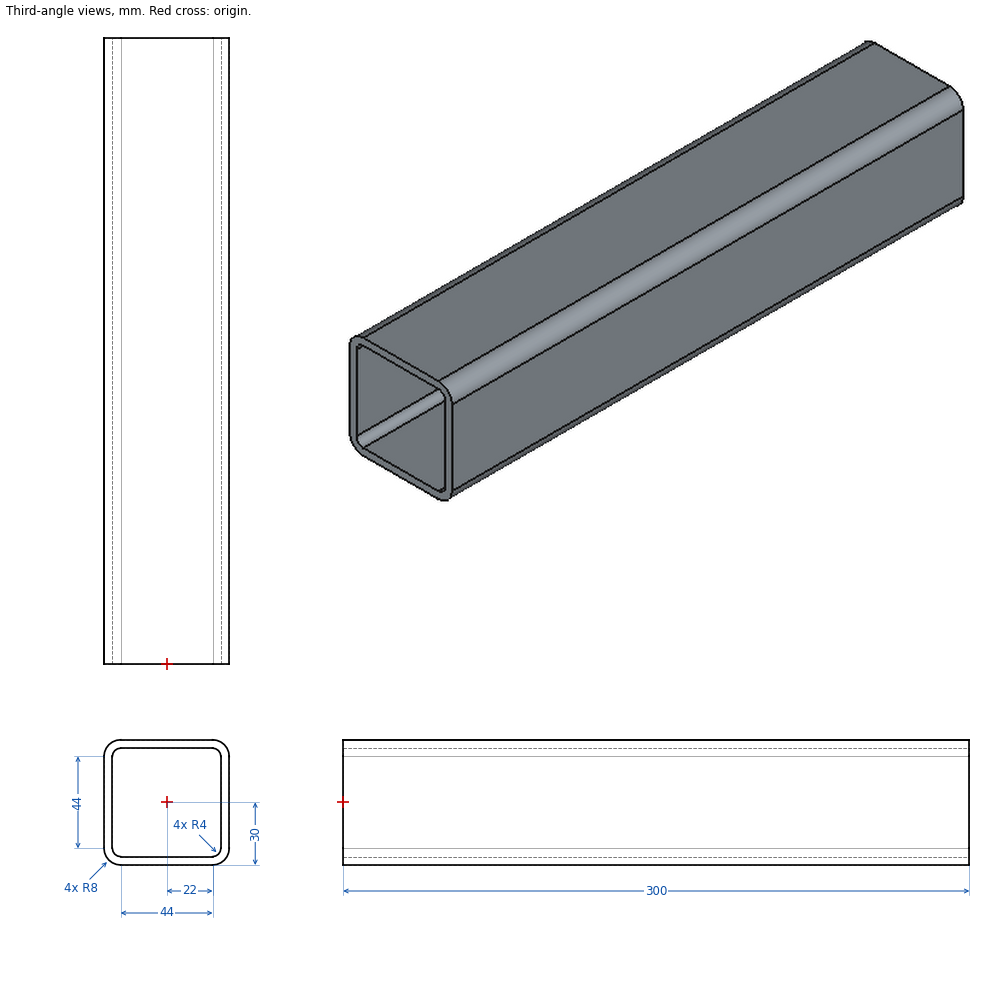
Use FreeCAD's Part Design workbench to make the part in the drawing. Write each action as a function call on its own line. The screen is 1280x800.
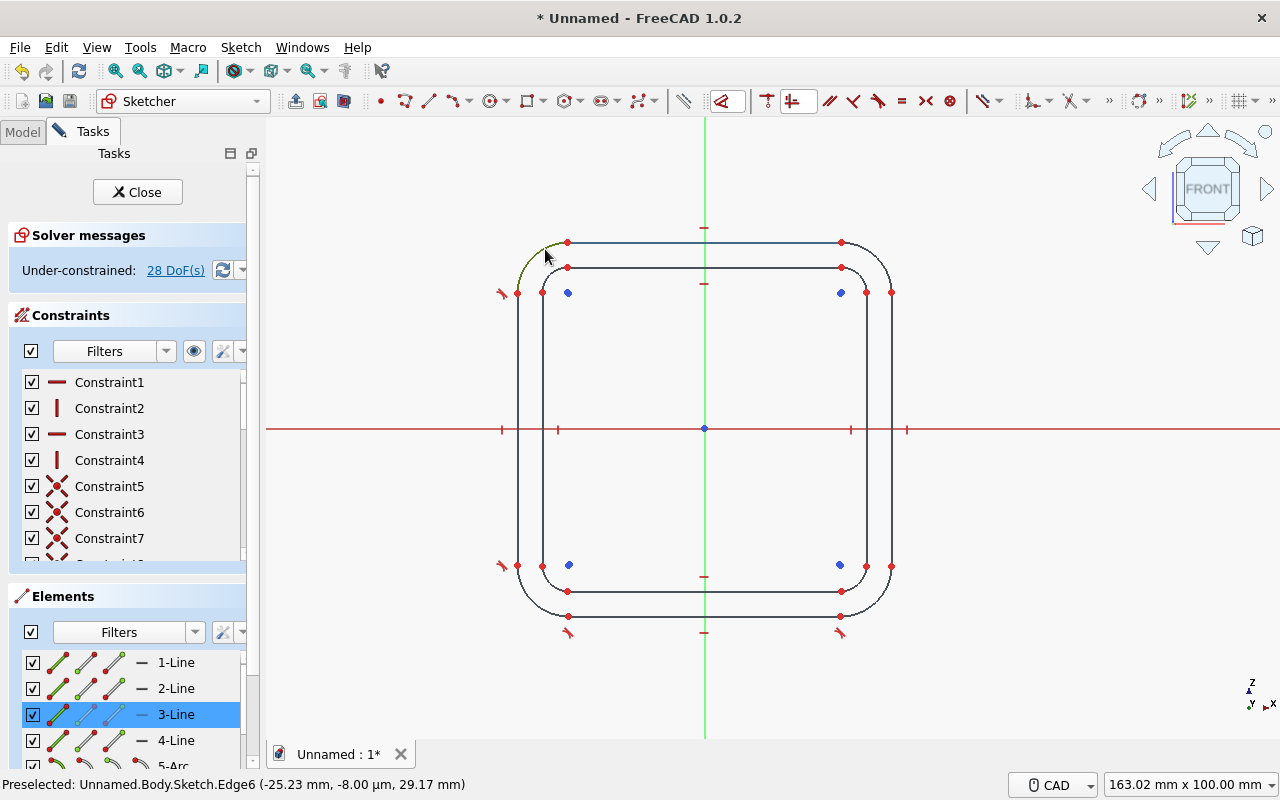
key(t)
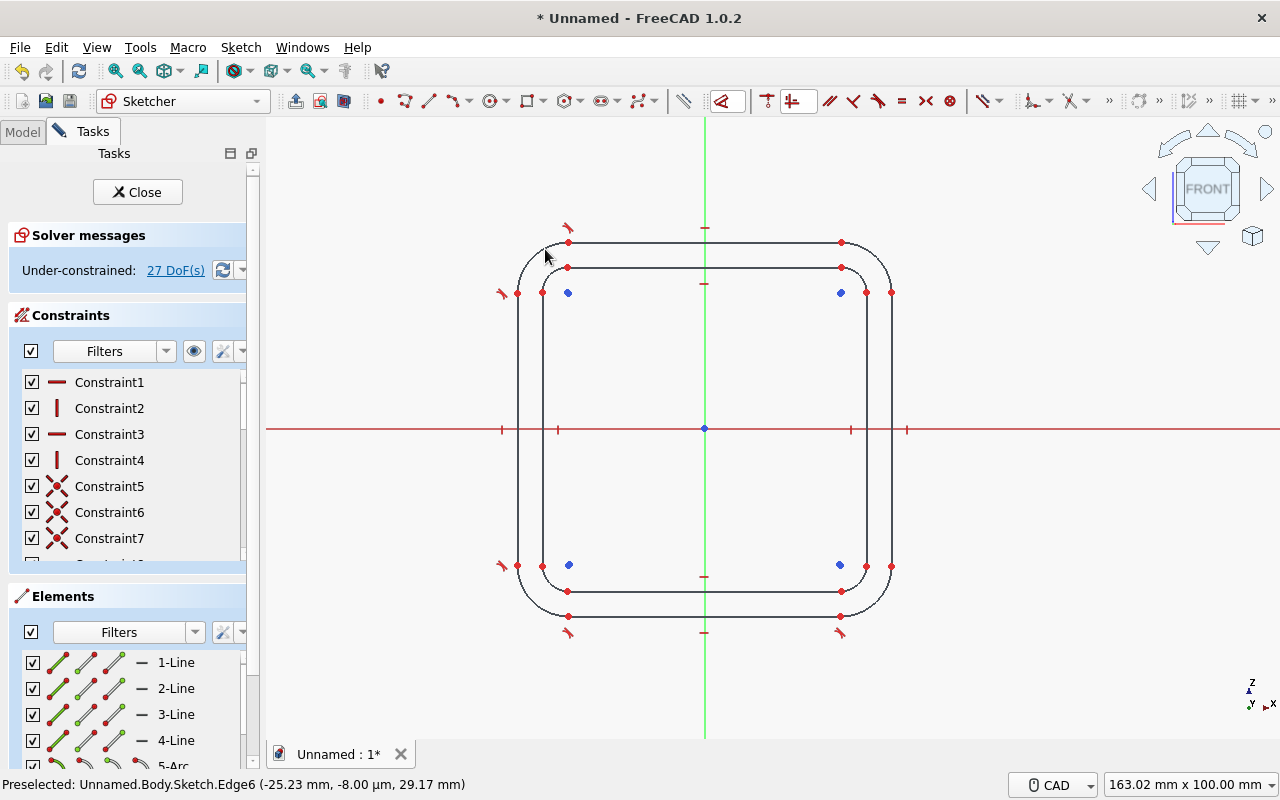
click(651, 243)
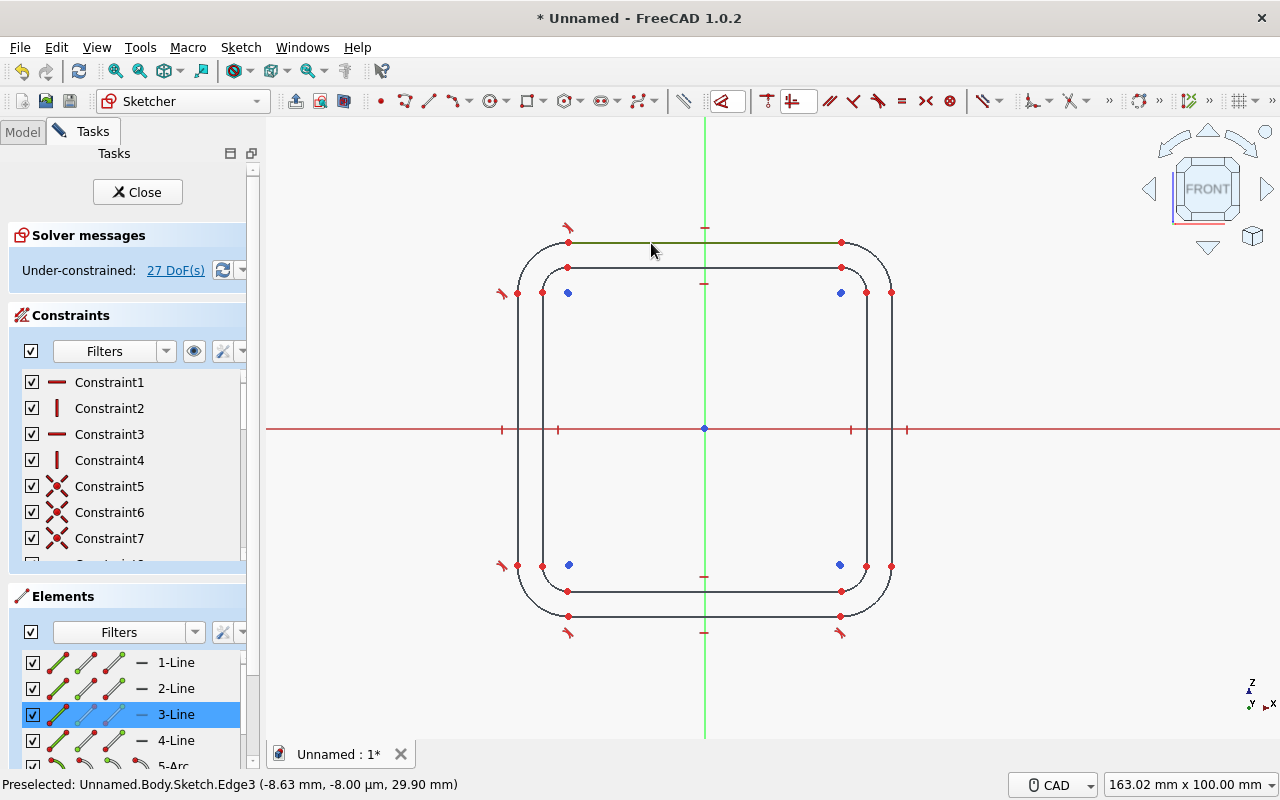
click(886, 270)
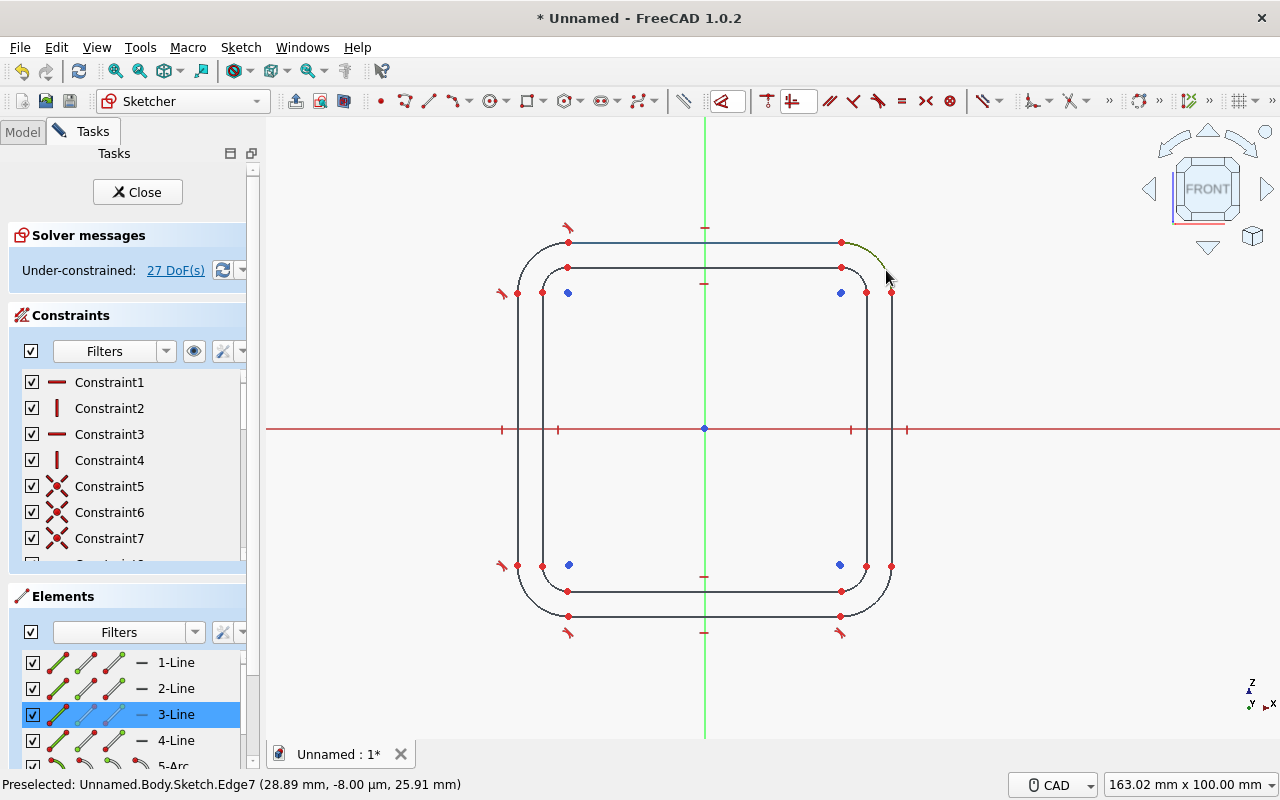
click(878, 102)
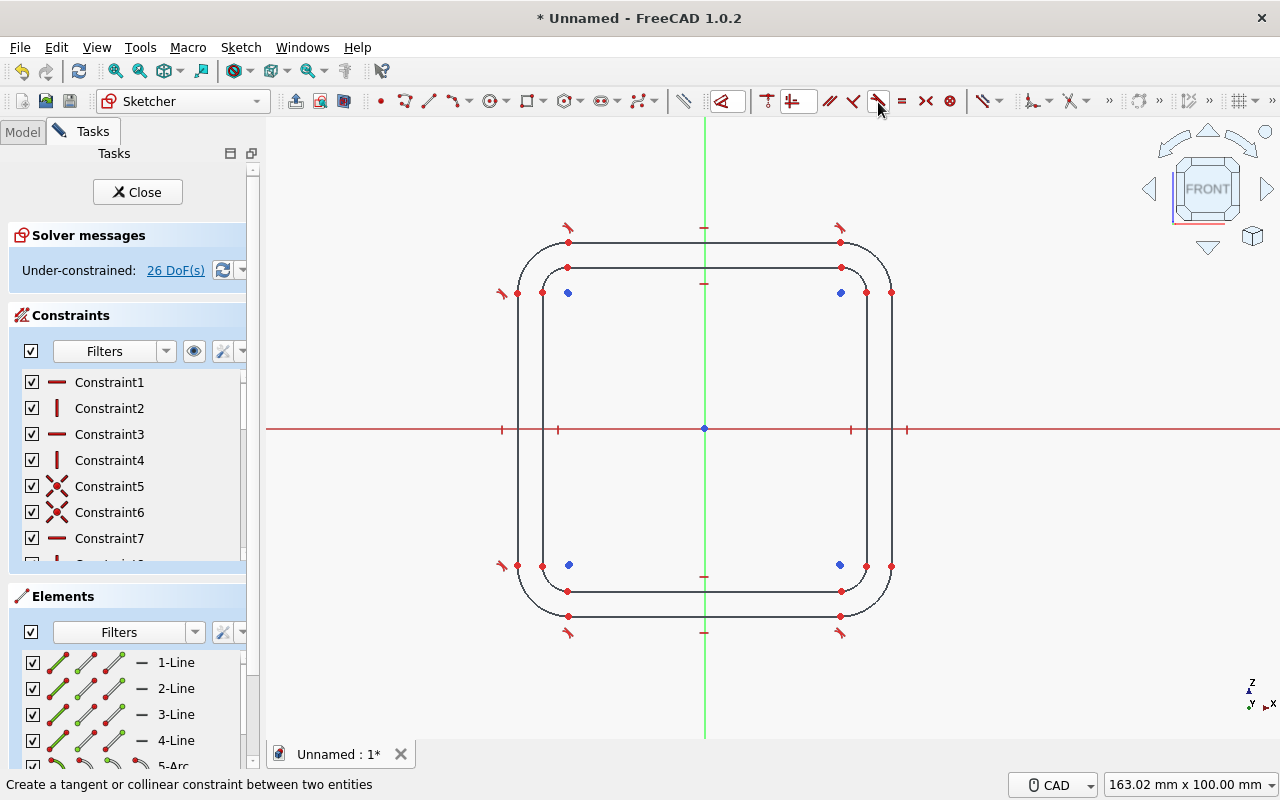
click(892, 375)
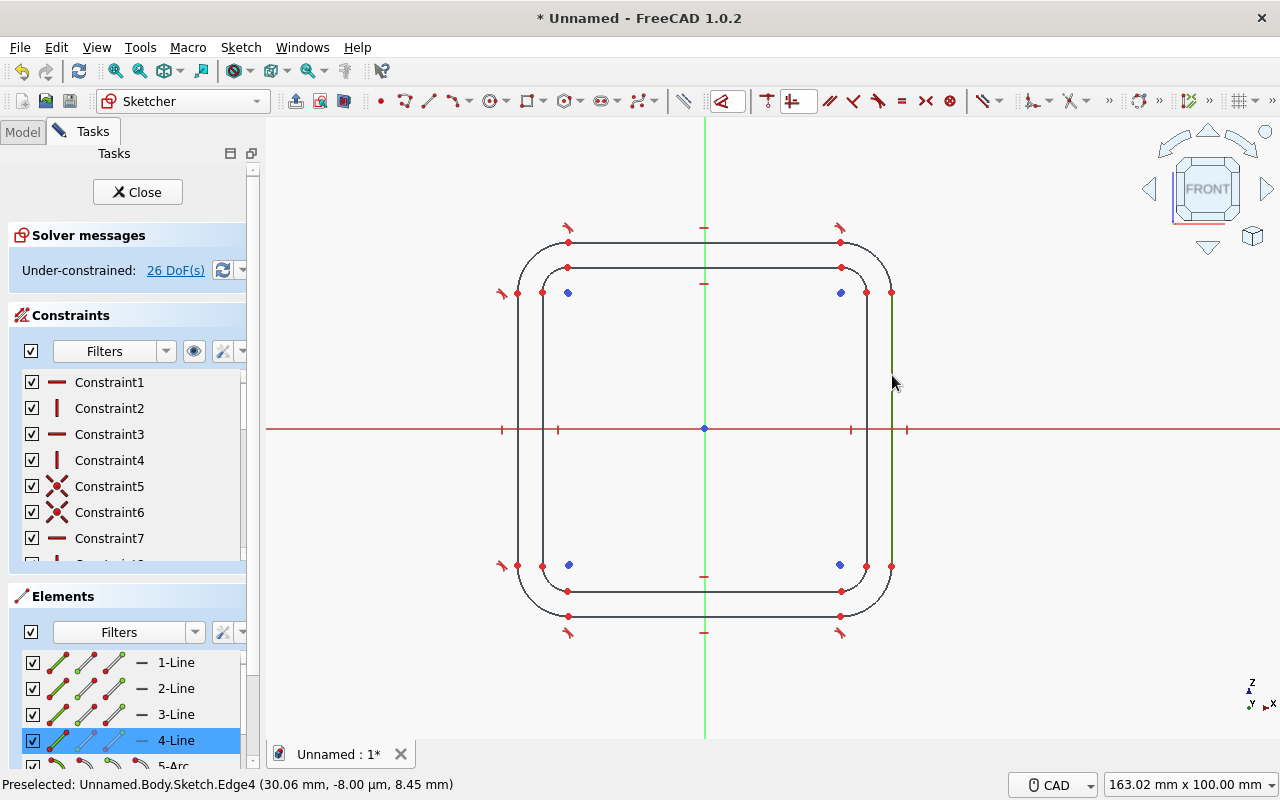
click(886, 270)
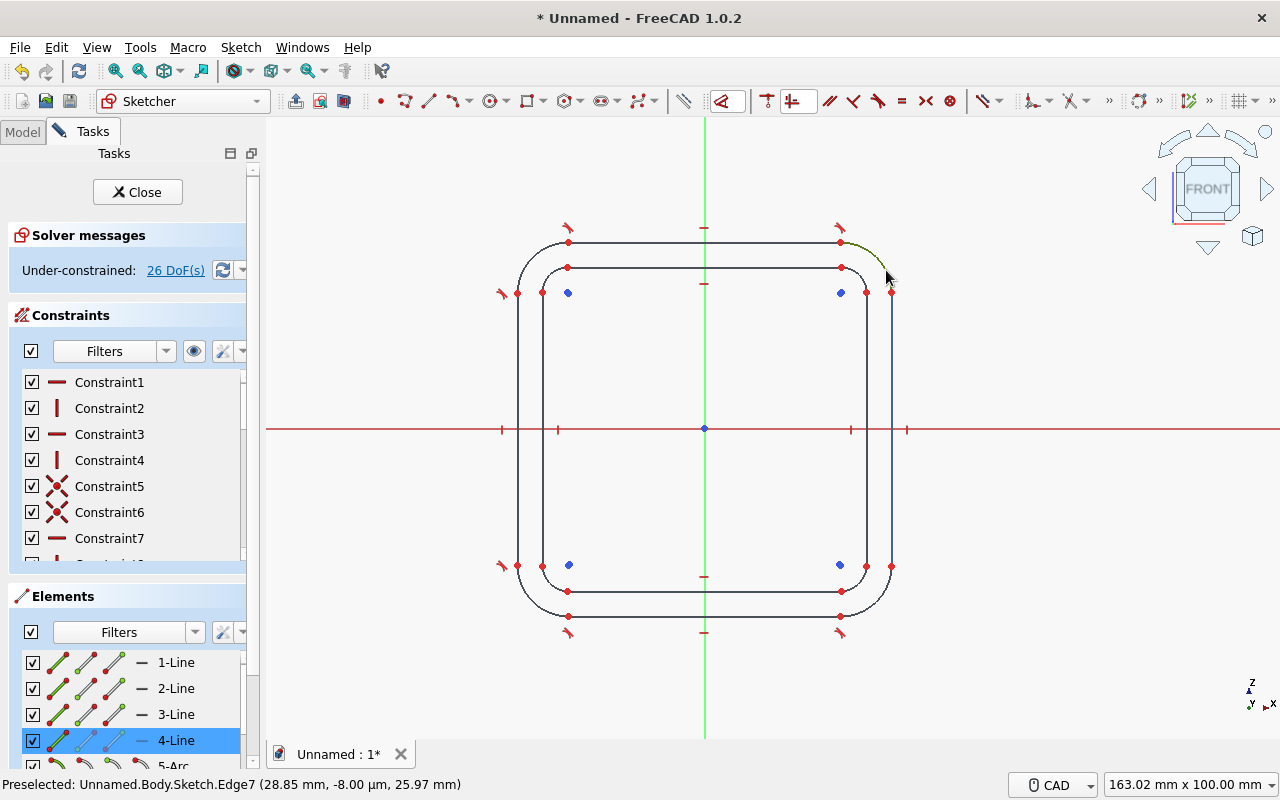
key(t)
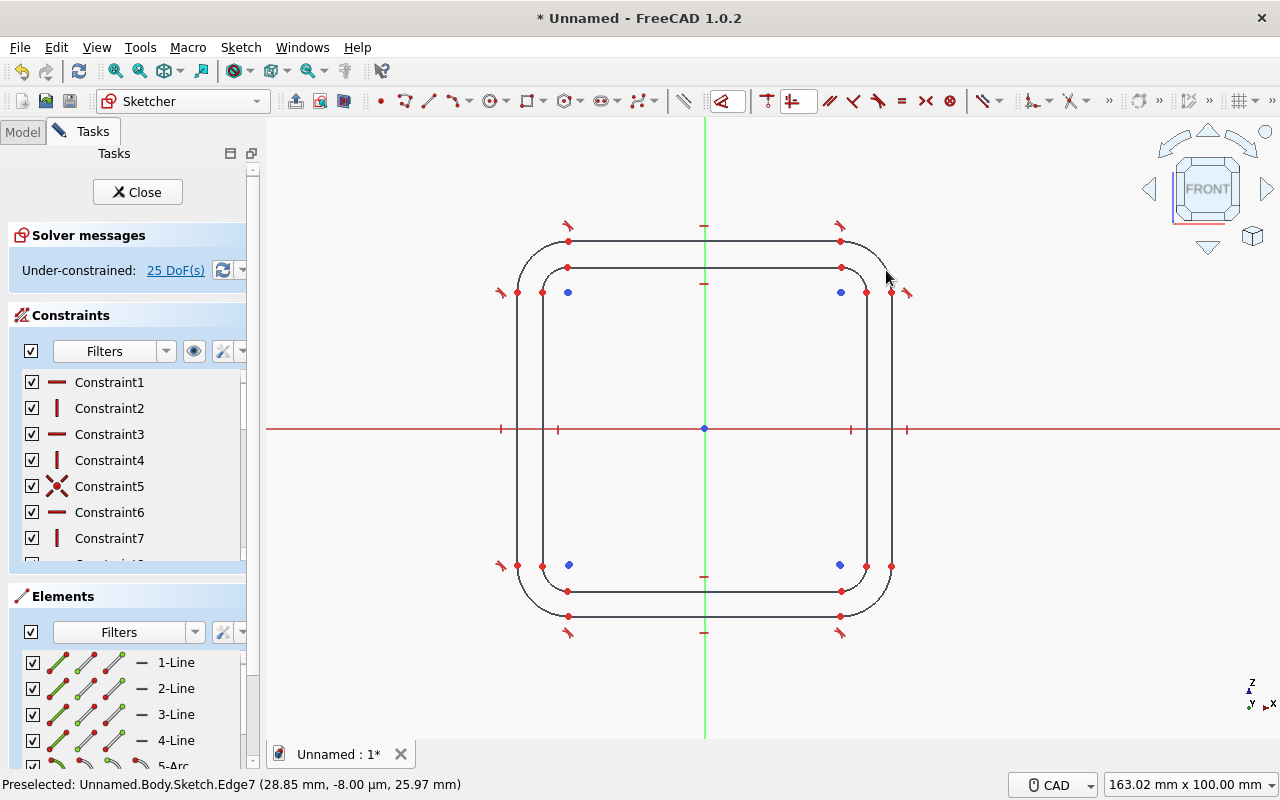
click(892, 375)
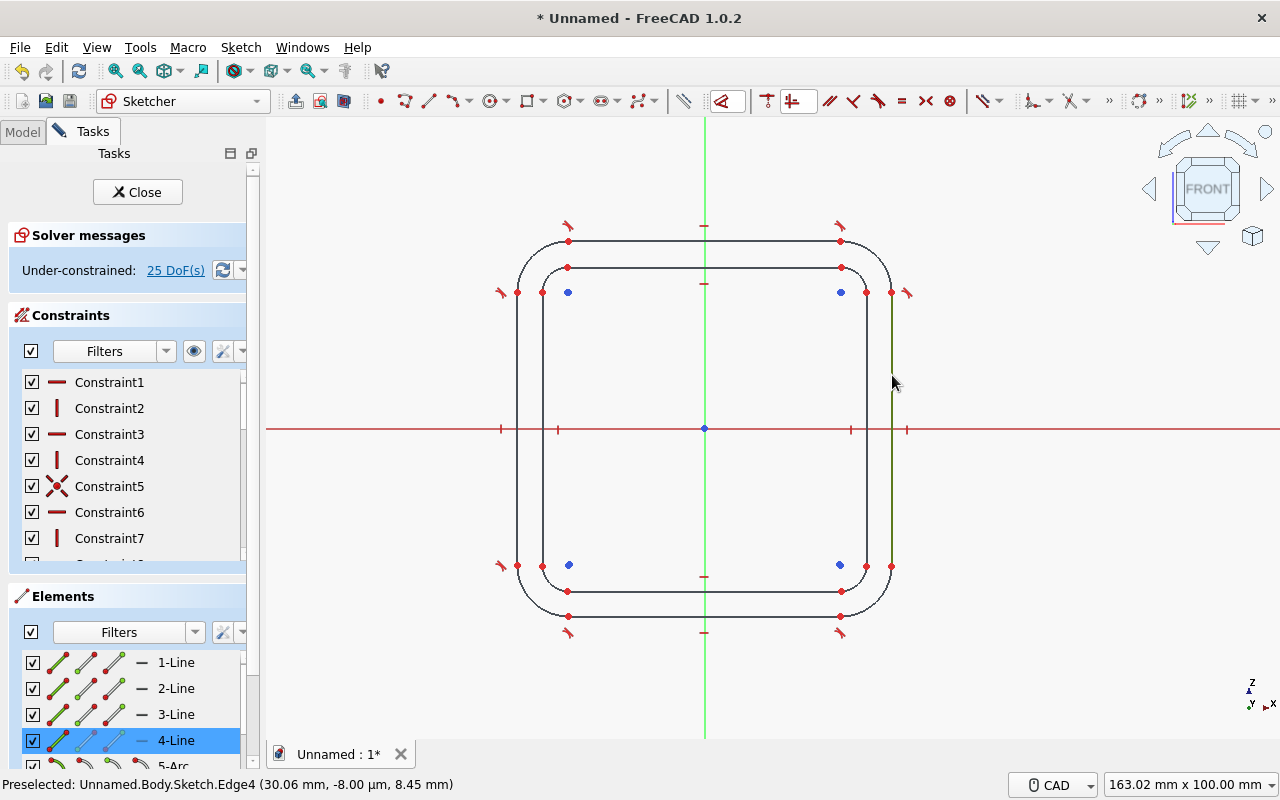
click(863, 611)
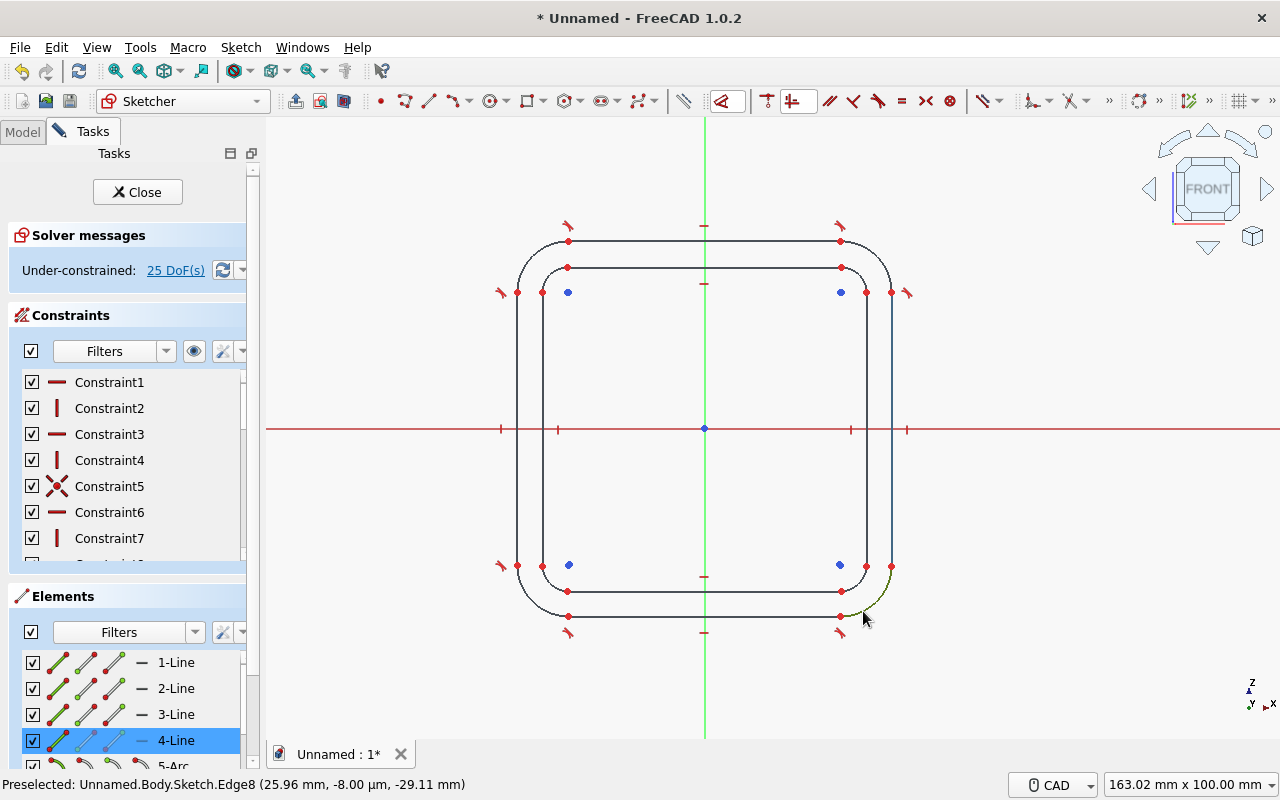
key(t)